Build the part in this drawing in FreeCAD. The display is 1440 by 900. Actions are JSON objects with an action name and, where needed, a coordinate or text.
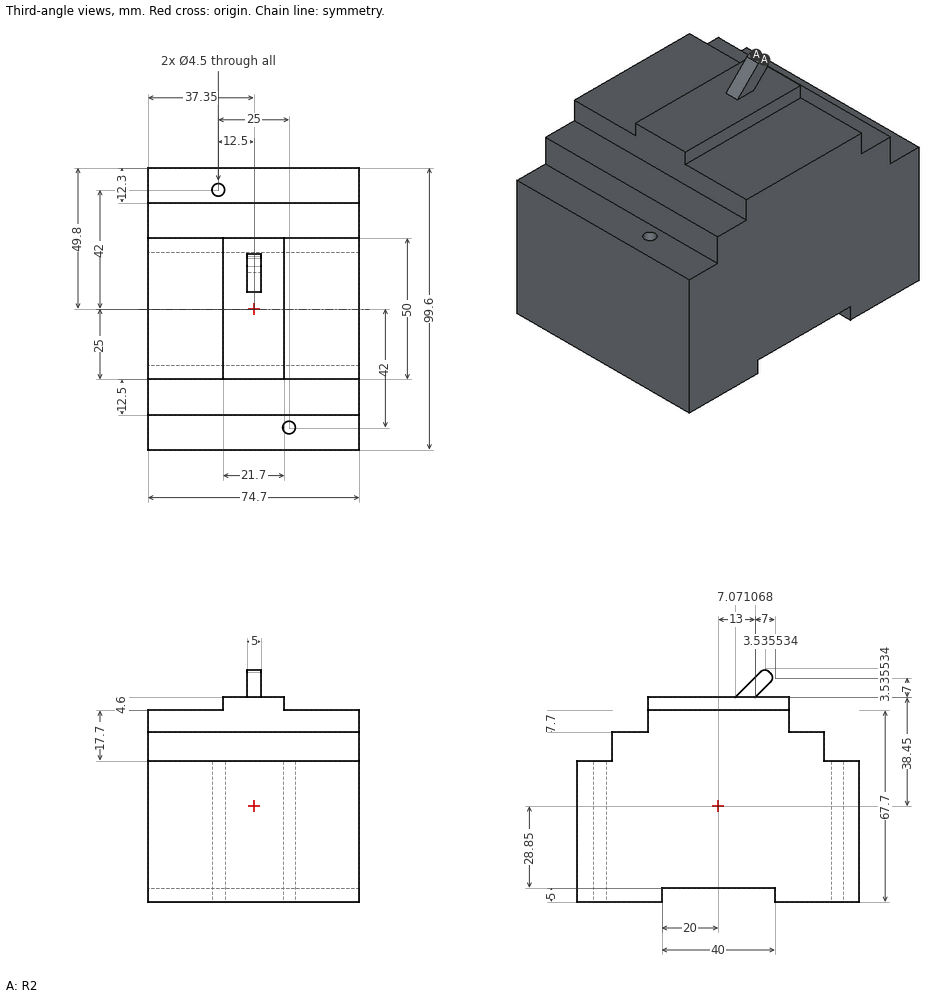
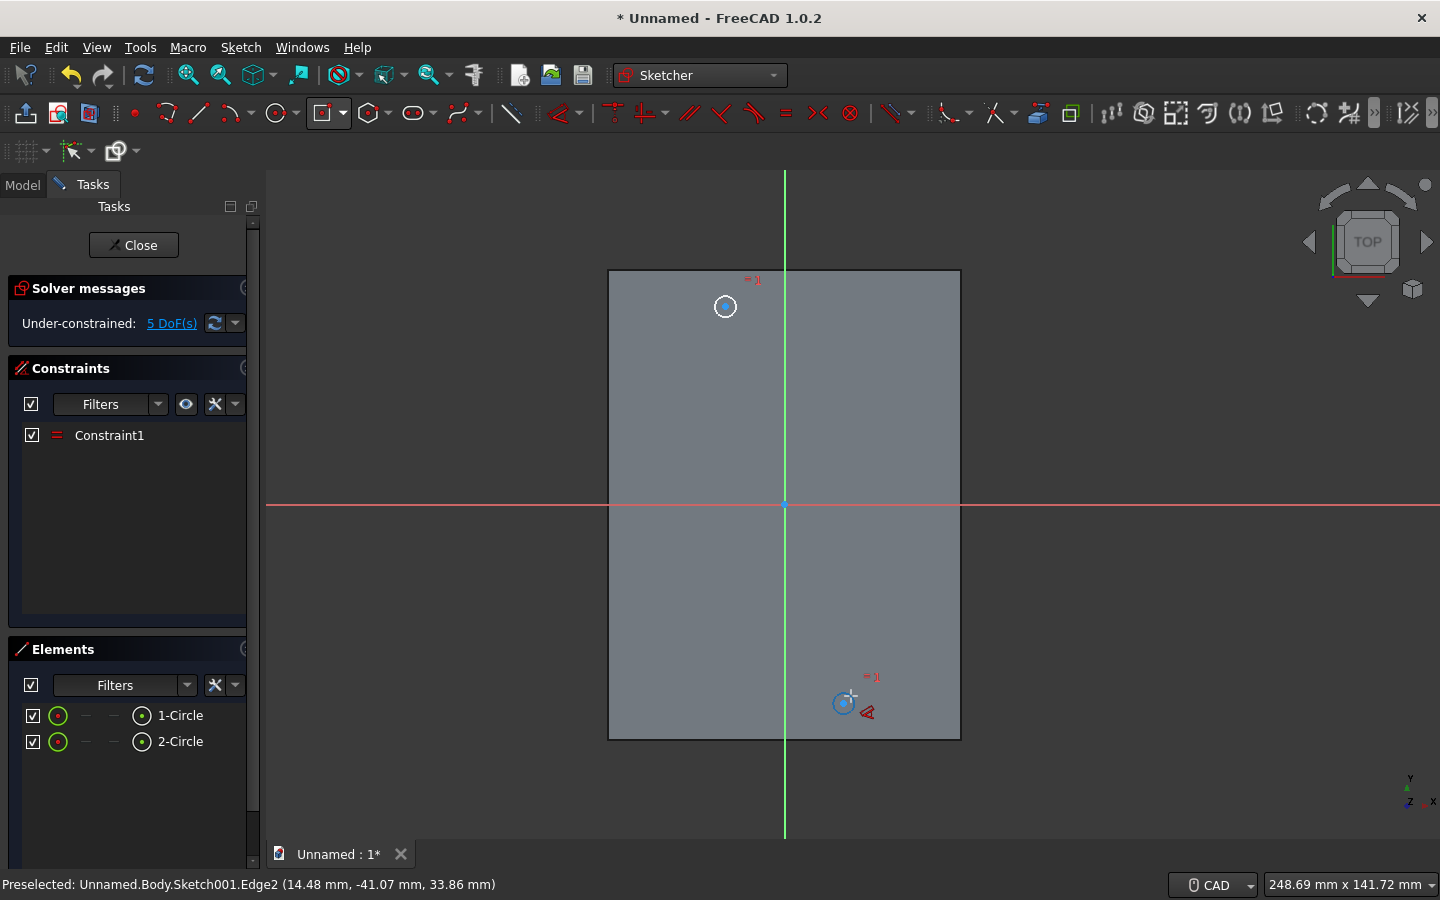
{"action": "scroll", "coordinate": [733, 299], "scroll_direction": "up", "scroll_amount": 4}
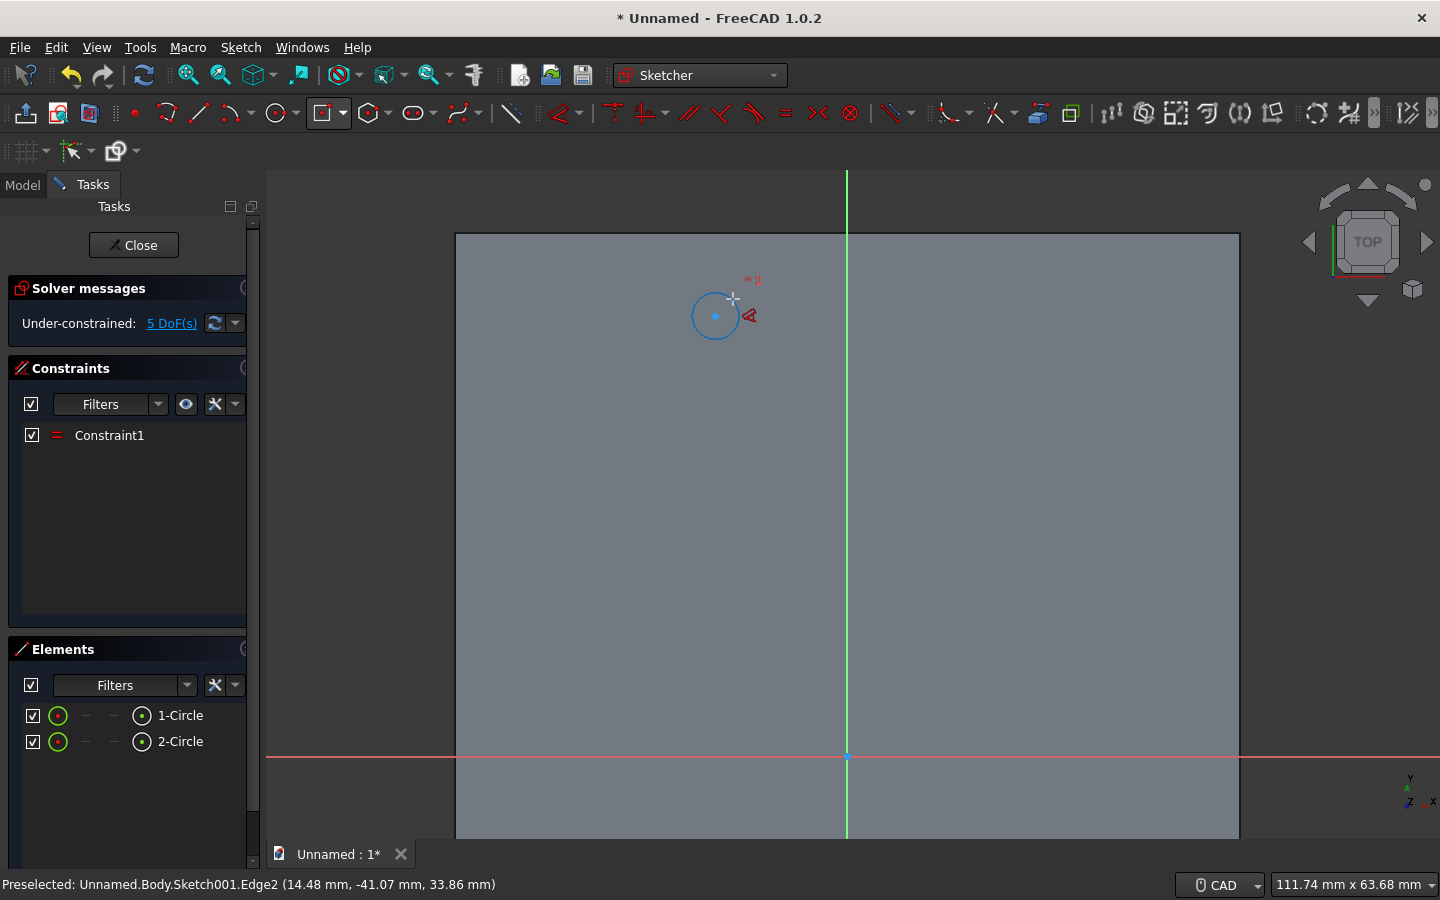
{"action": "left_click", "coordinate": [732, 300]}
{"action": "left_click", "coordinate": [755, 278]}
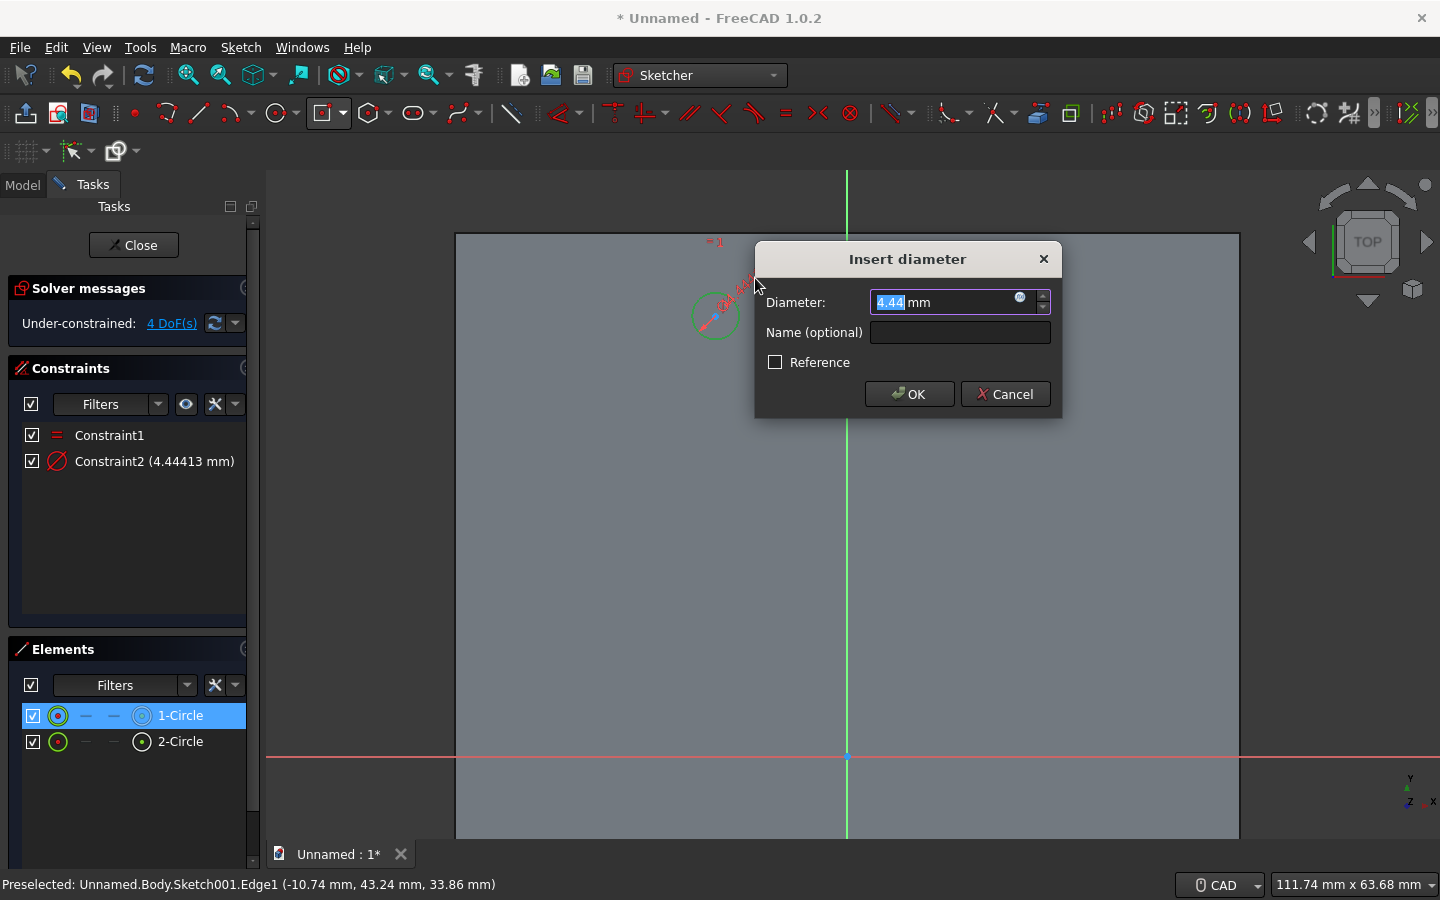
{"action": "type", "text": "4.5"}
{"action": "key", "text": "Return"}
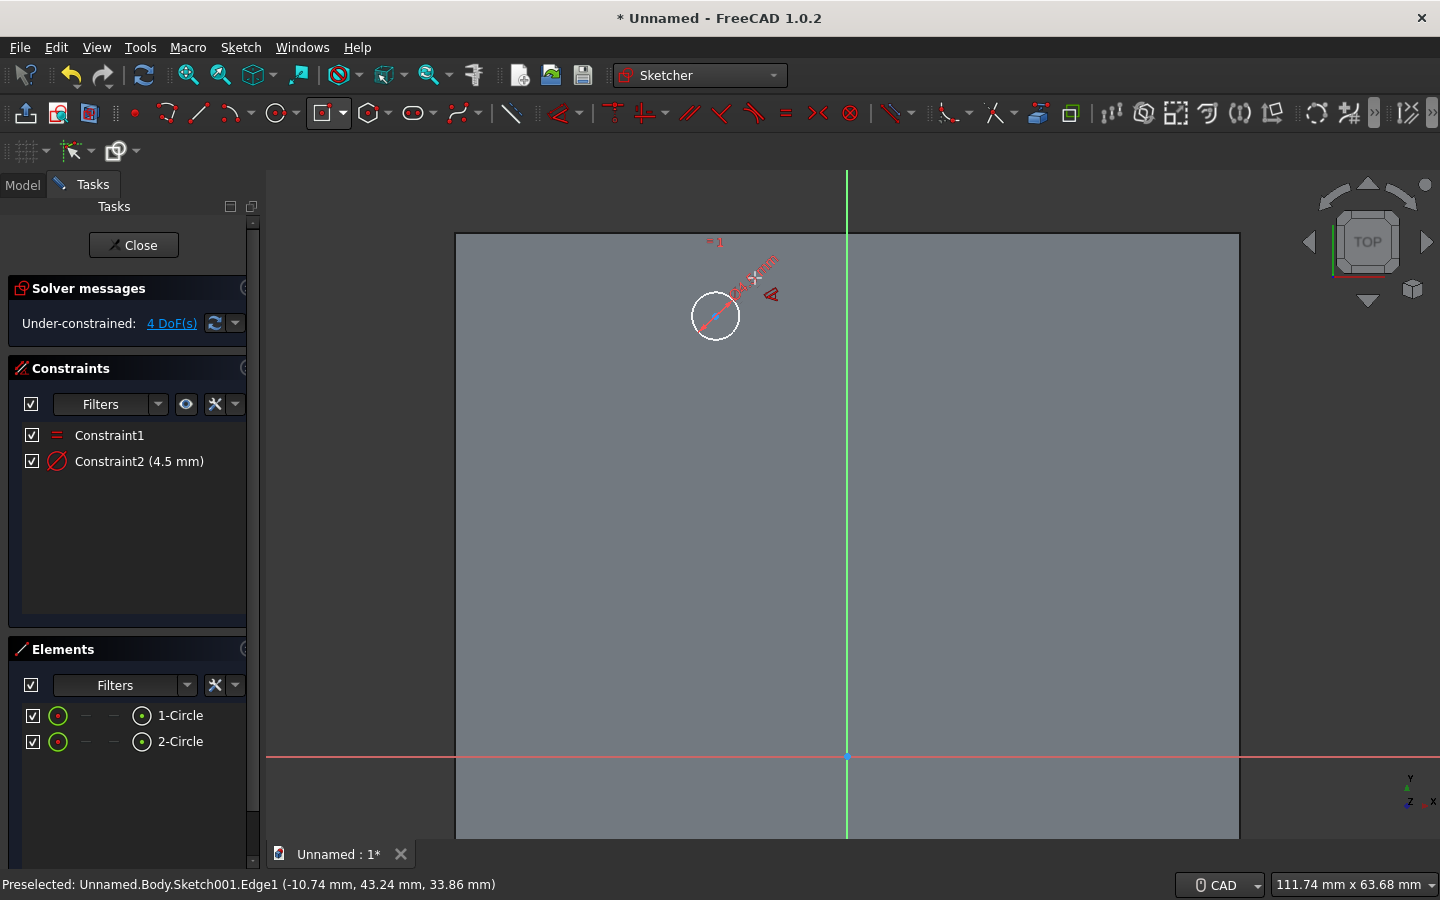
{"action": "left_click", "coordinate": [716, 316]}
{"action": "left_click", "coordinate": [682, 536]}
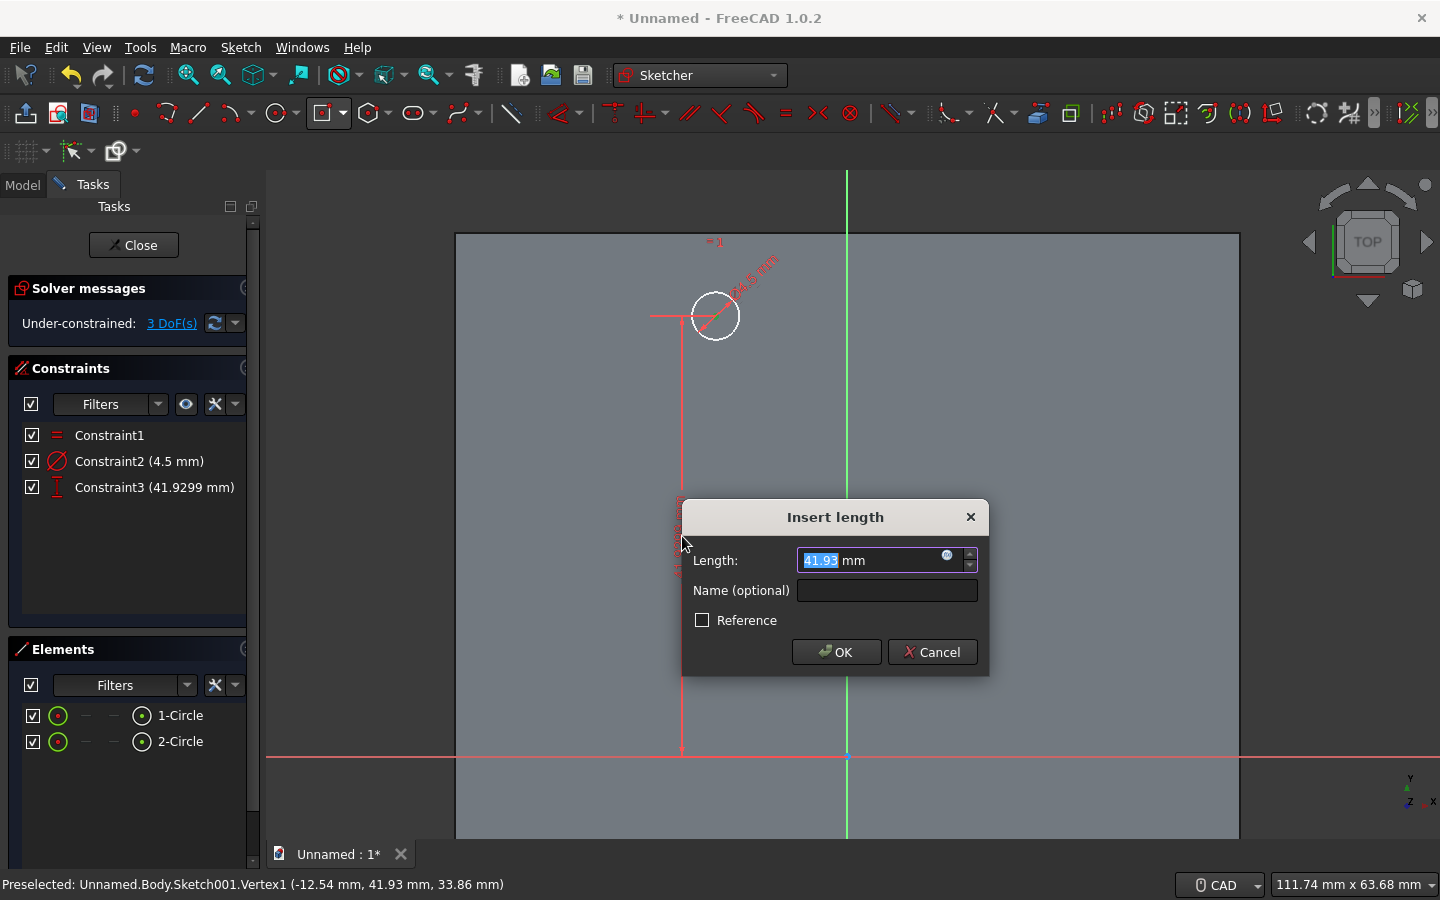
{"action": "type", "text": "42"}
{"action": "key", "text": "Return"}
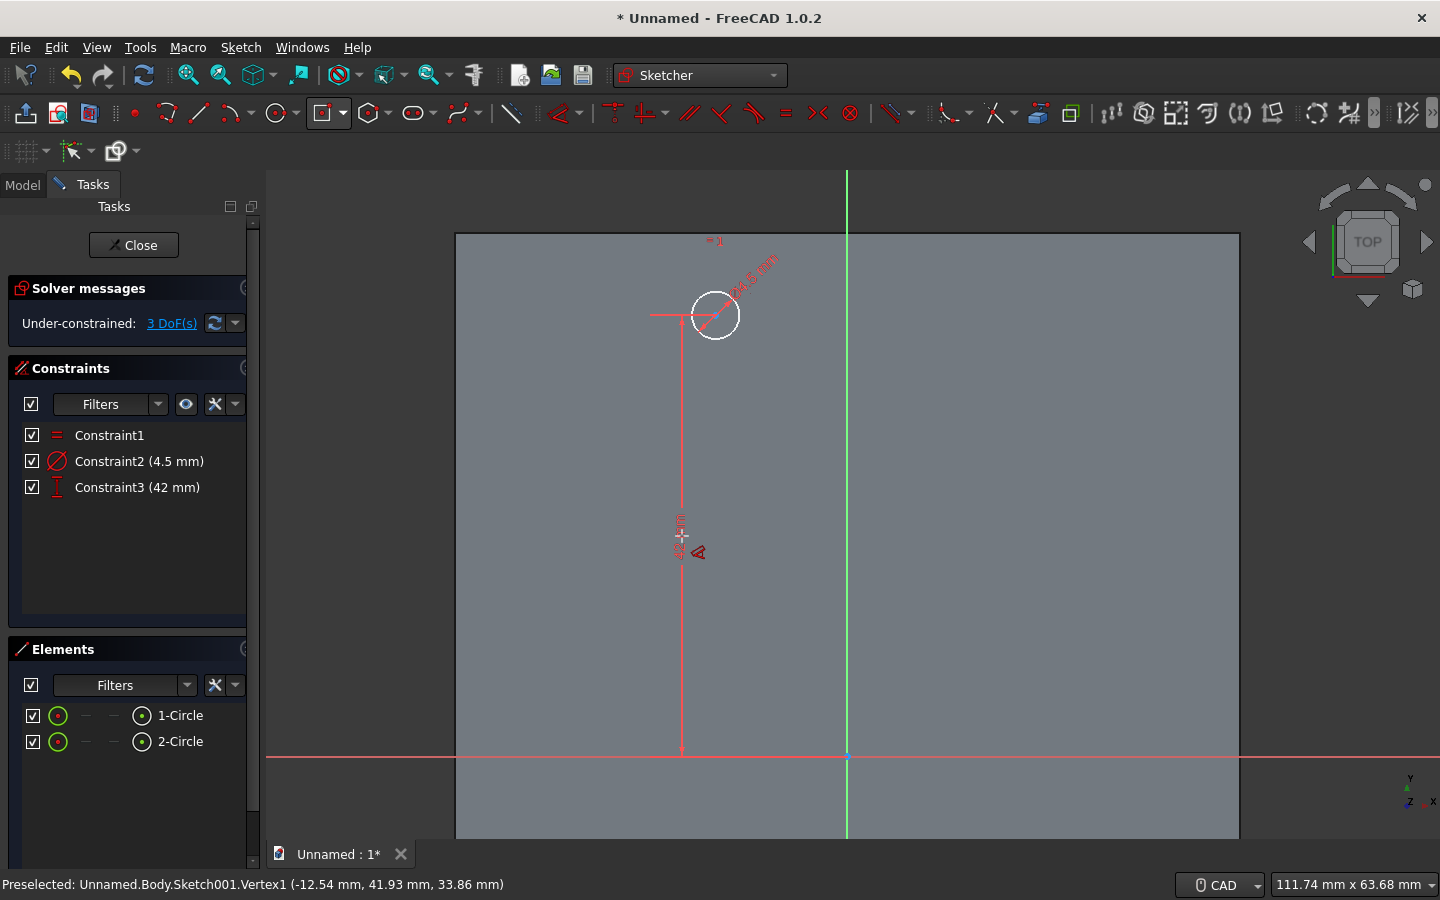
{"action": "scroll", "coordinate": [733, 299], "scroll_direction": "down", "scroll_amount": 4}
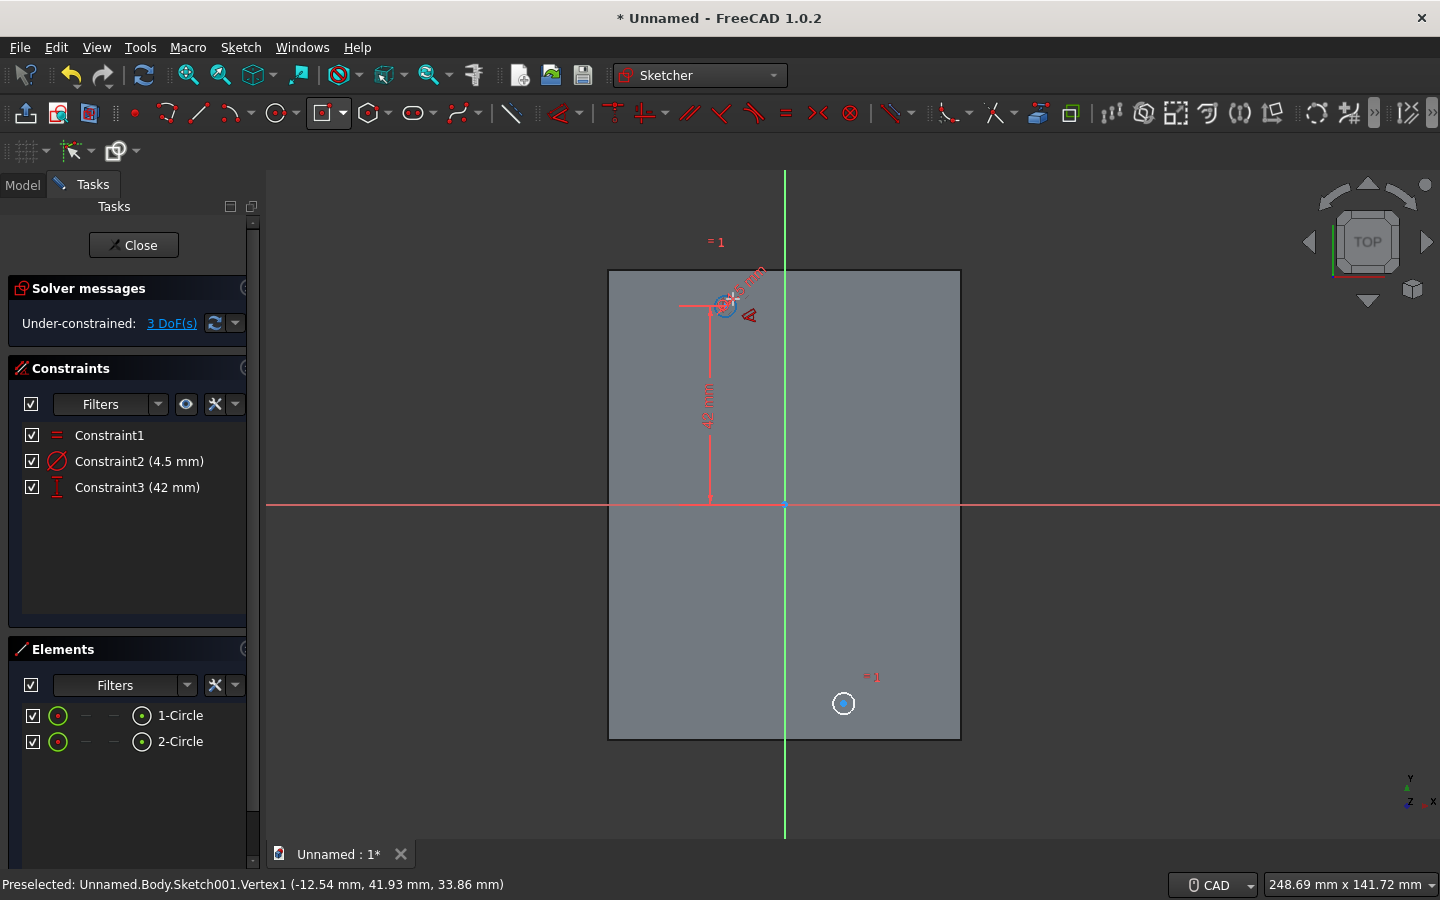
{"action": "left_click", "coordinate": [844, 704]}
{"action": "left_click", "coordinate": [878, 604]}